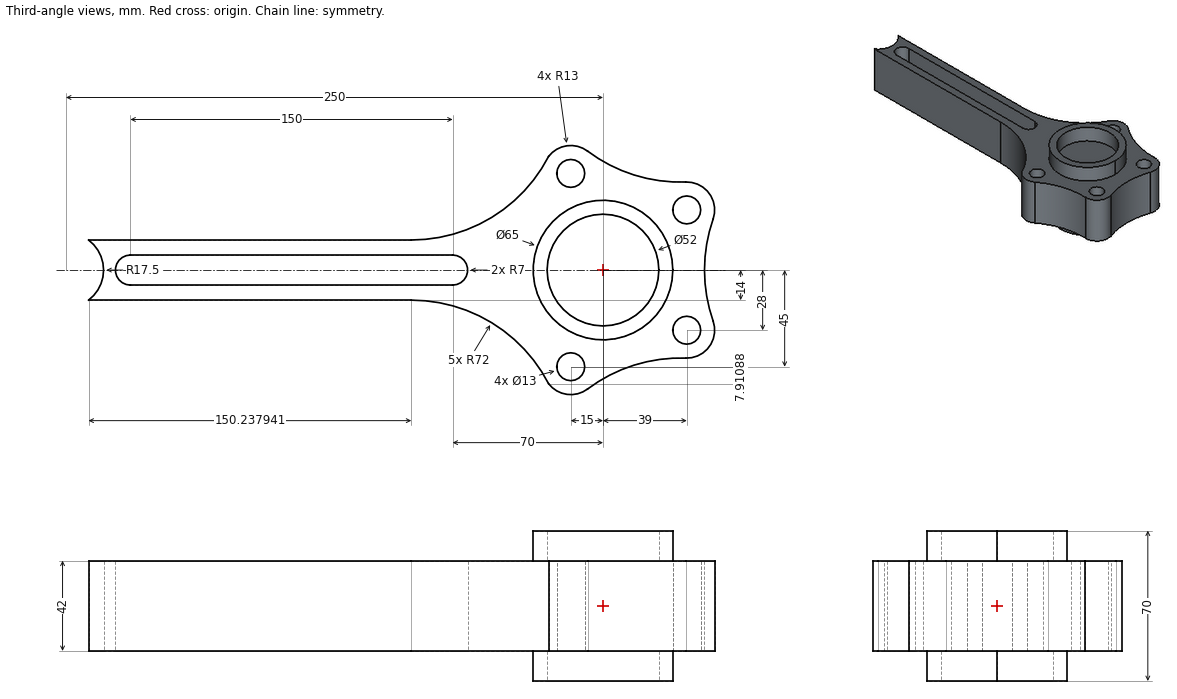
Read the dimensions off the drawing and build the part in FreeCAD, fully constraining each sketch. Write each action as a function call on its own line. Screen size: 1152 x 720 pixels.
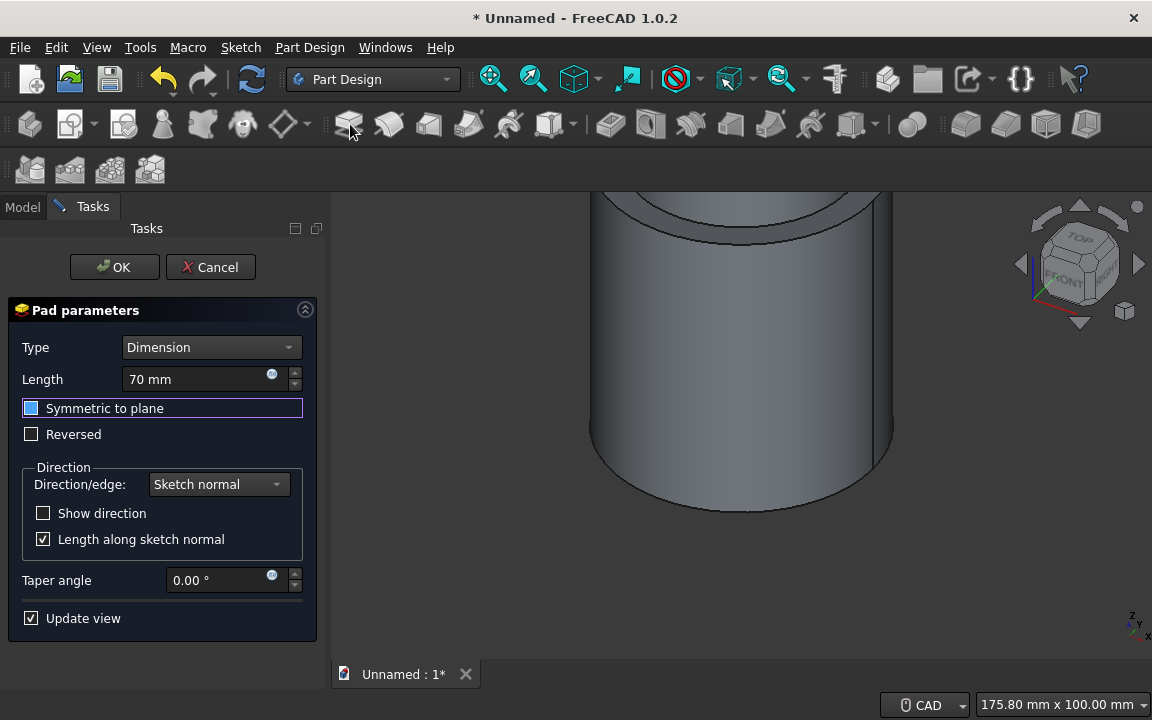
click(30, 408)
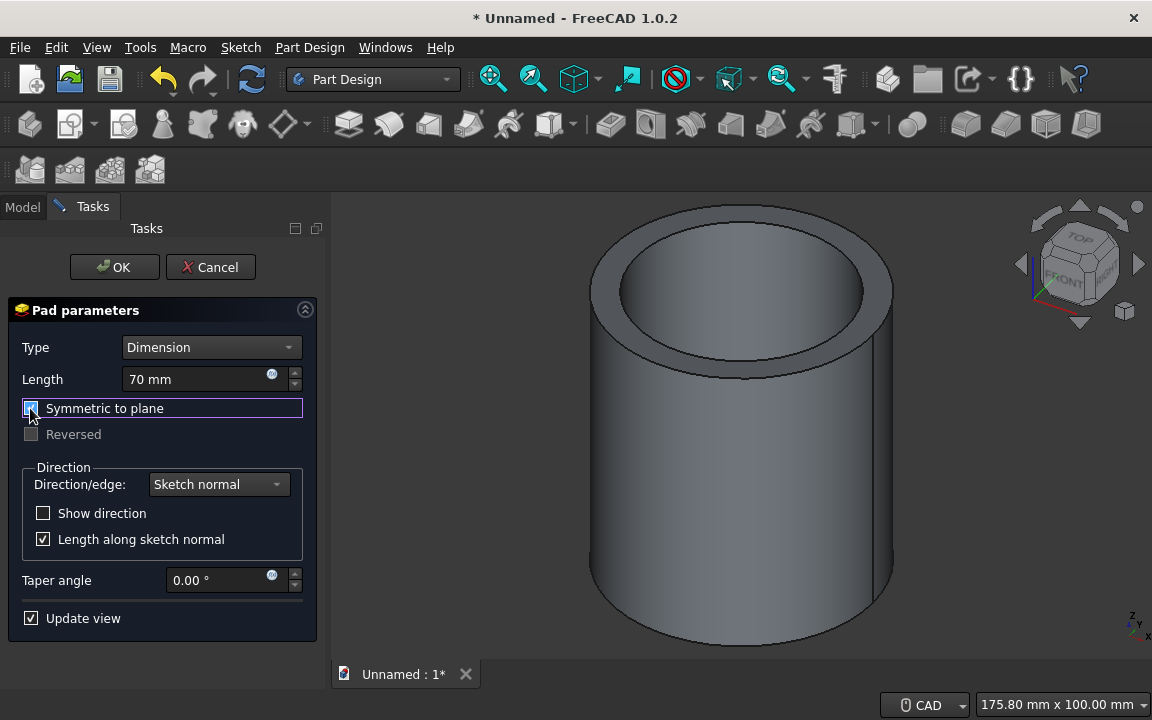
click(115, 267)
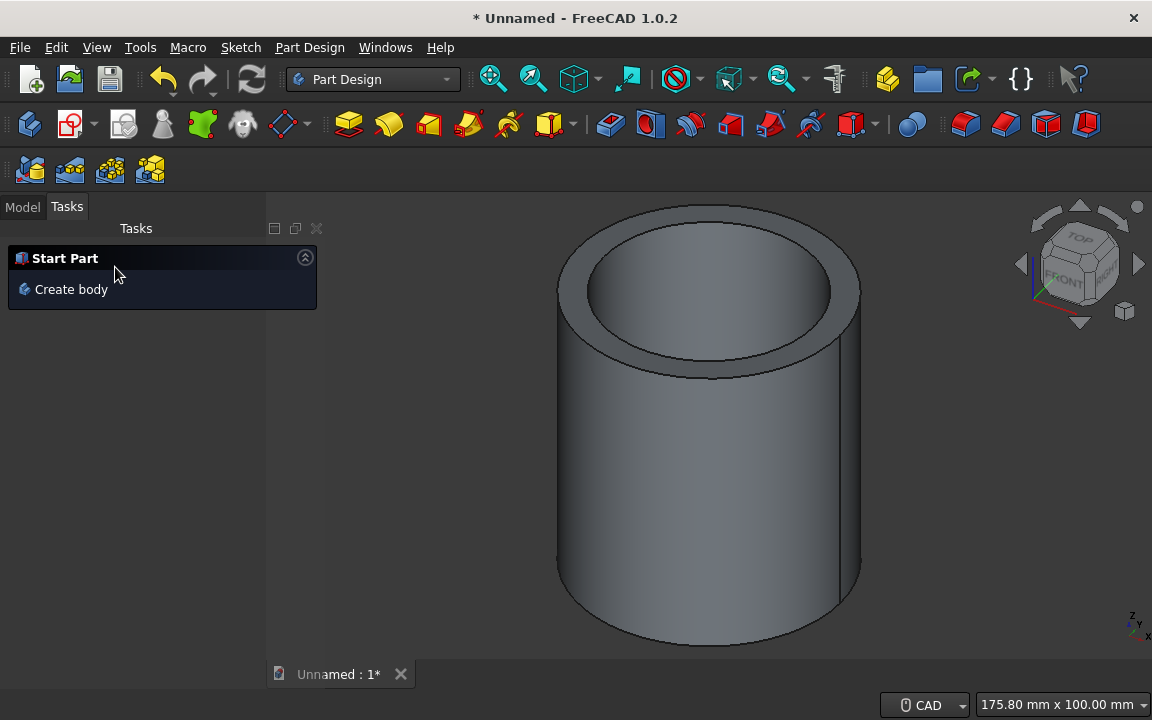
click(494, 80)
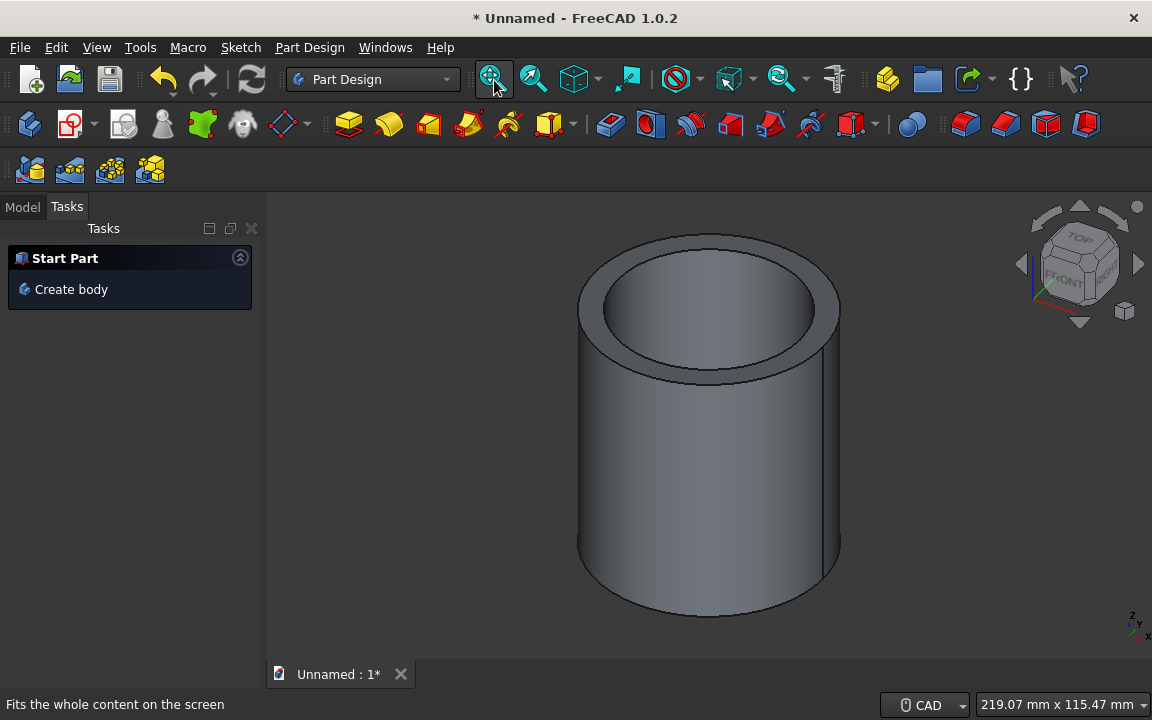
click(23, 206)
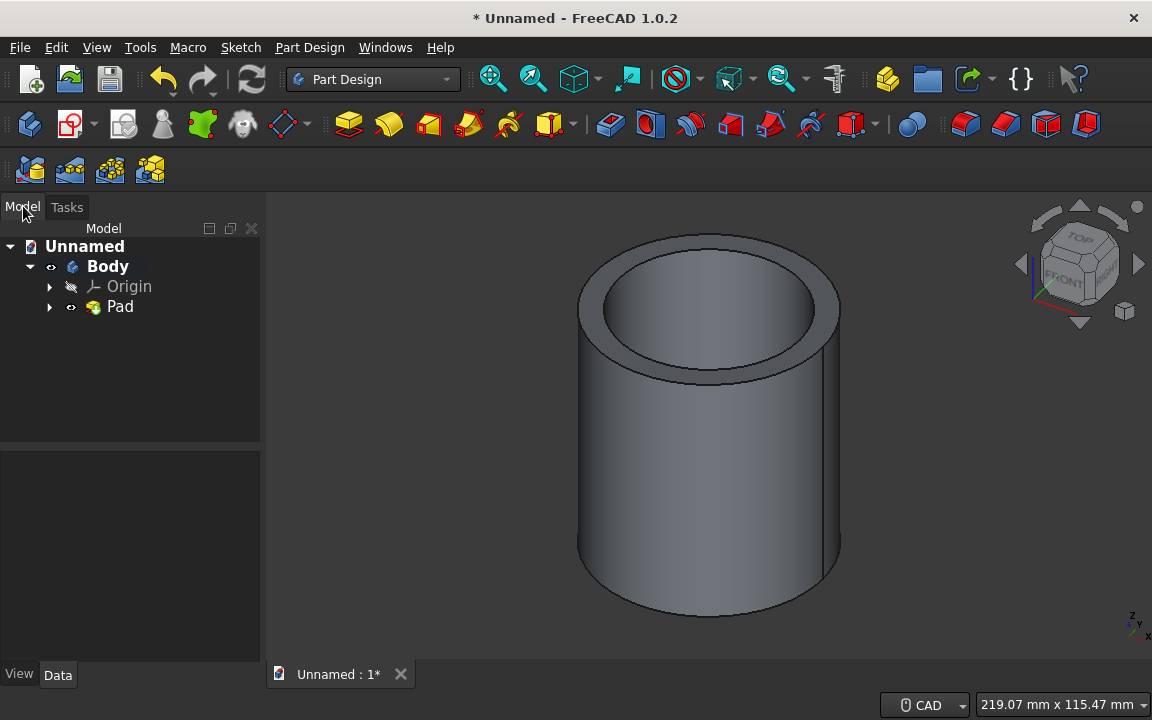
click(50, 287)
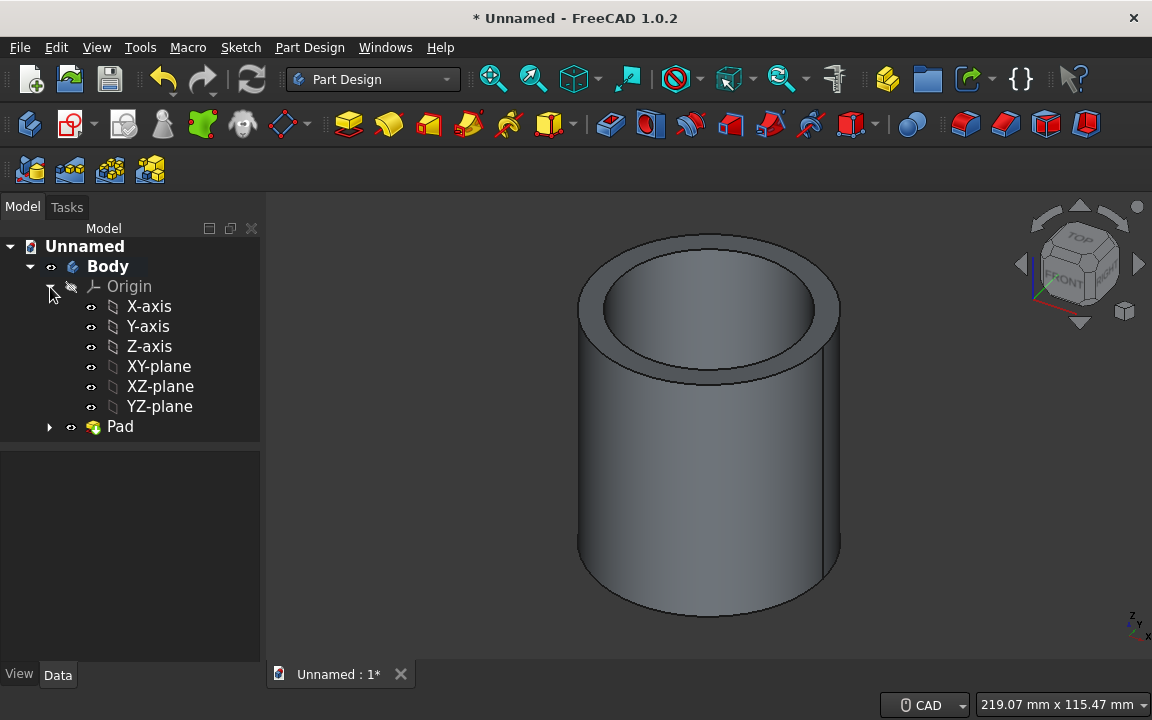
click(136, 367)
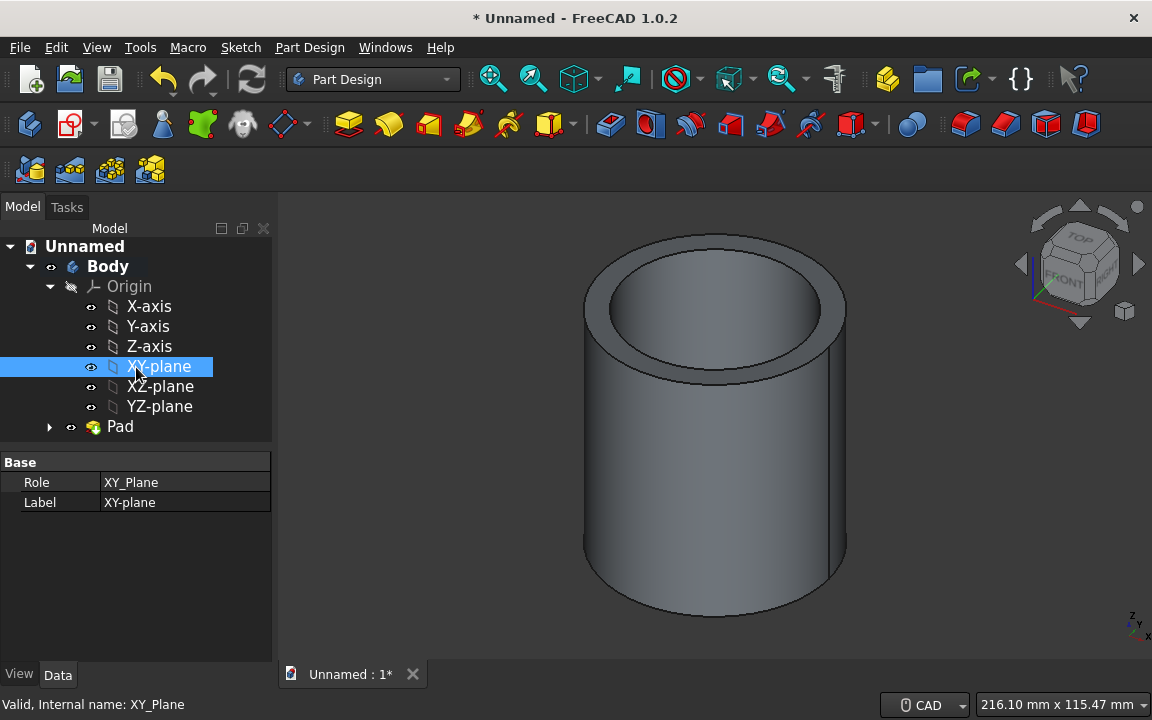
click(284, 124)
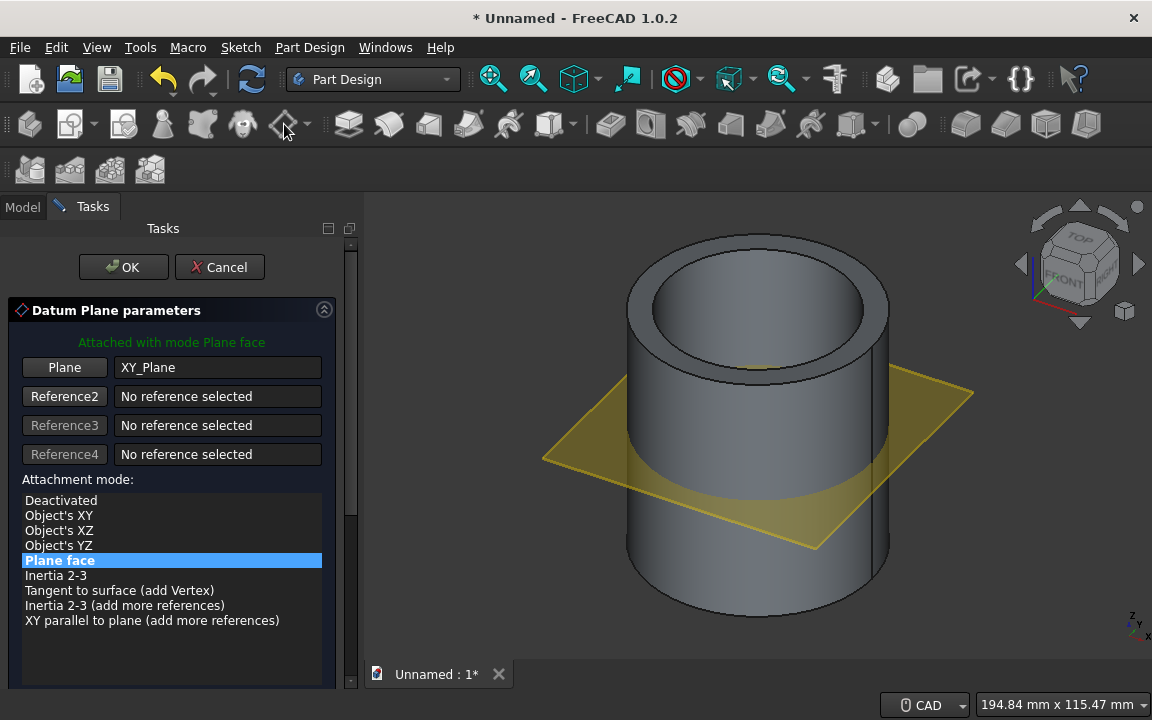
scroll(351, 463, down, 3)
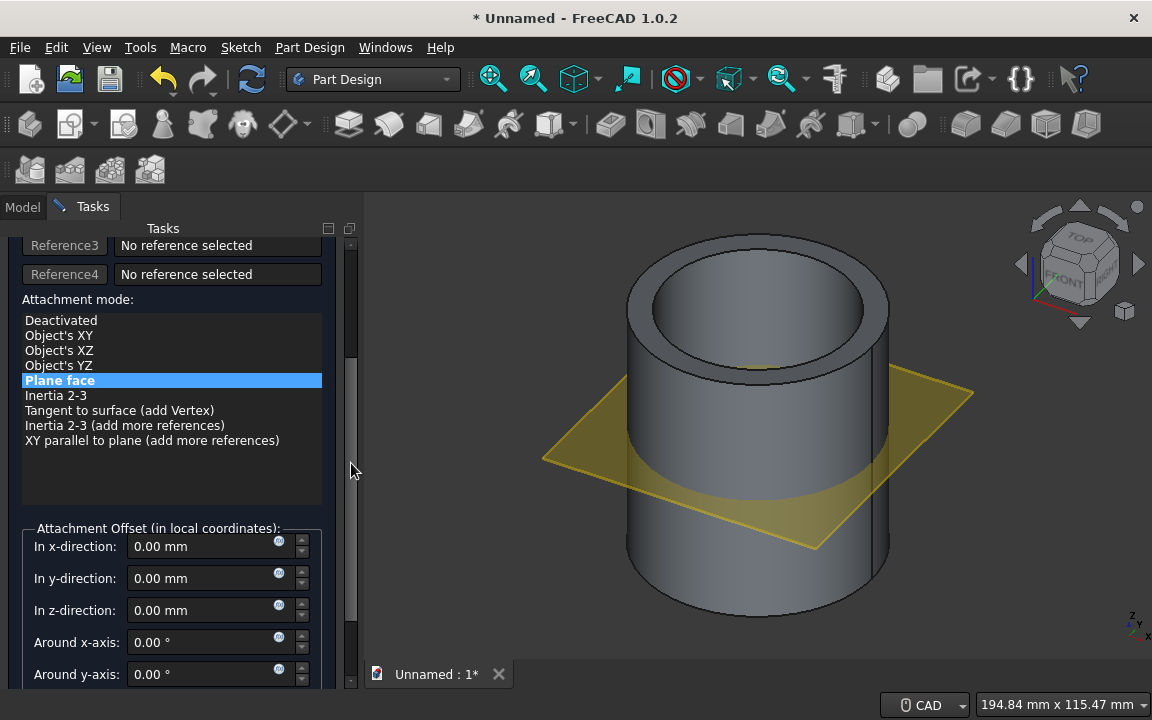
triple_click(210, 610)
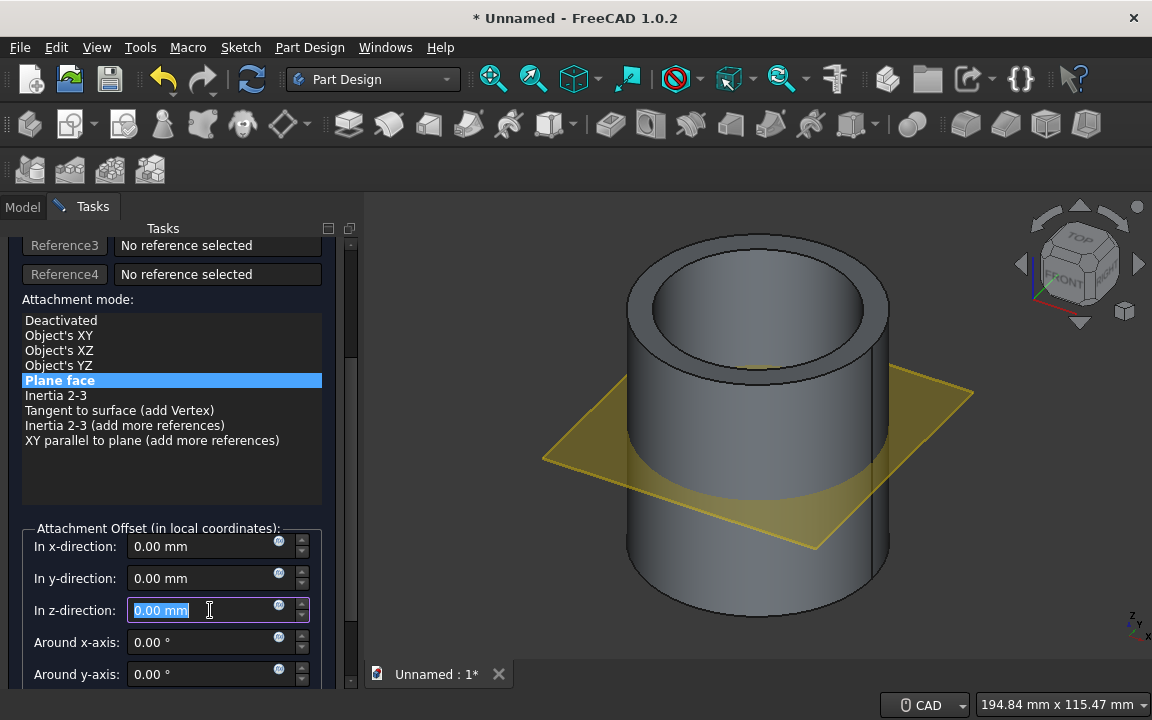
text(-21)
key(Tab)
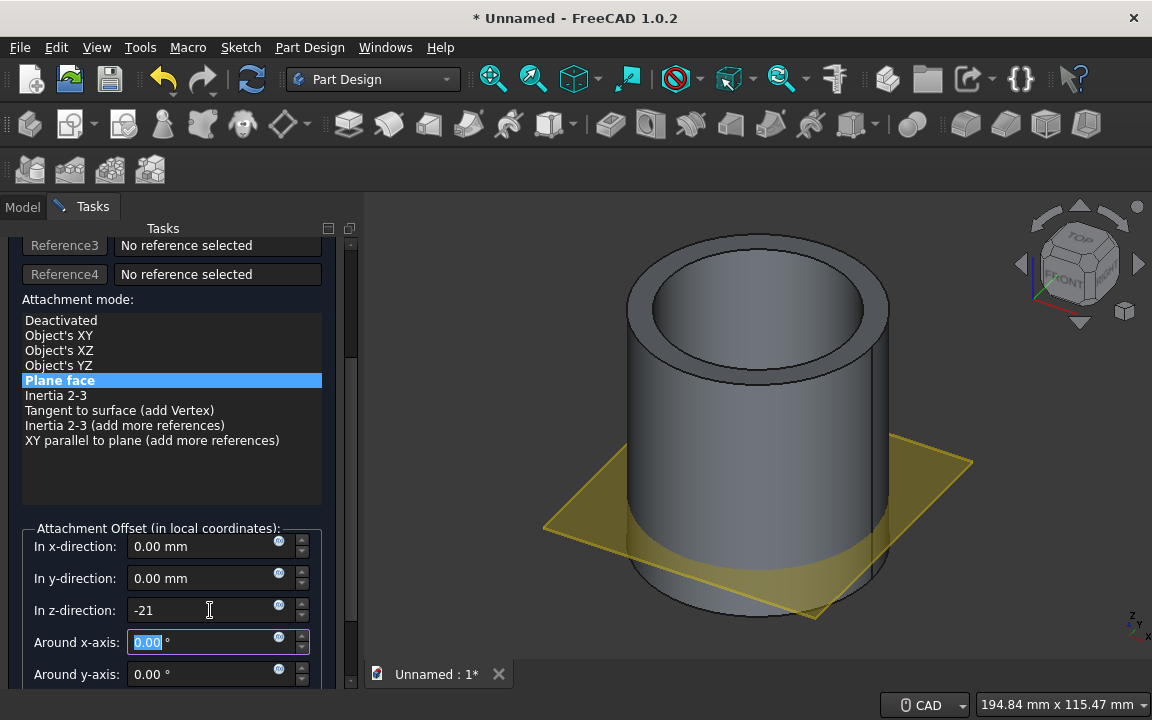
scroll(351, 463, up, 4)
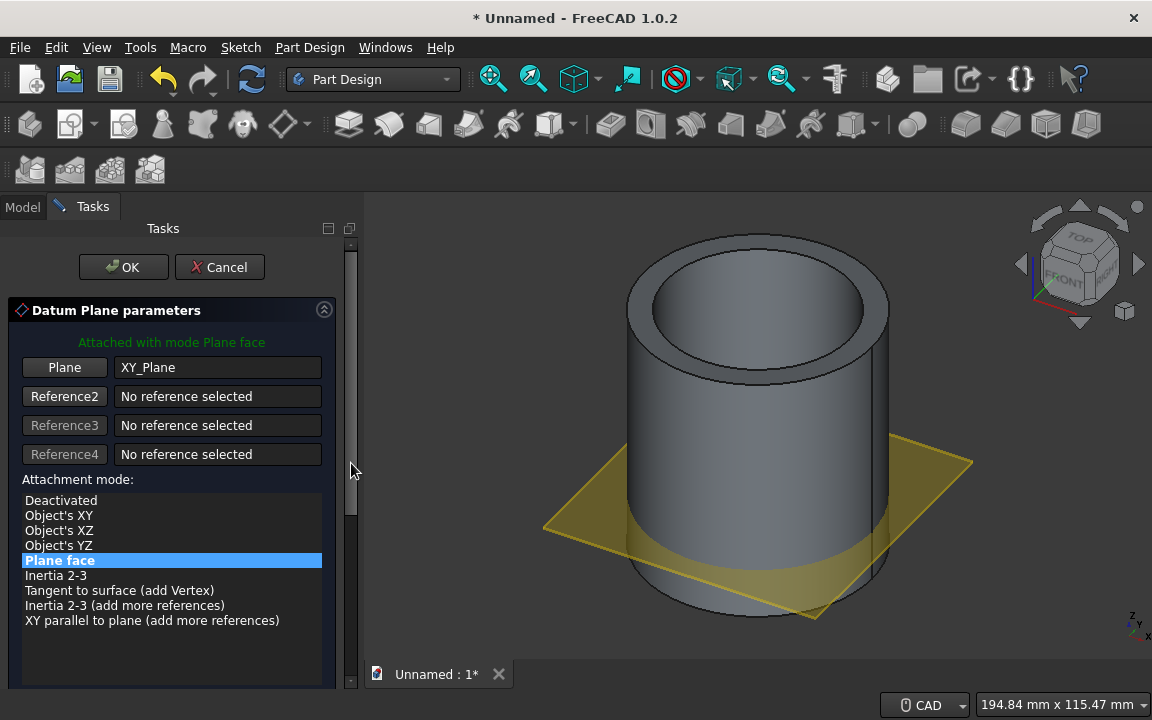
click(124, 267)